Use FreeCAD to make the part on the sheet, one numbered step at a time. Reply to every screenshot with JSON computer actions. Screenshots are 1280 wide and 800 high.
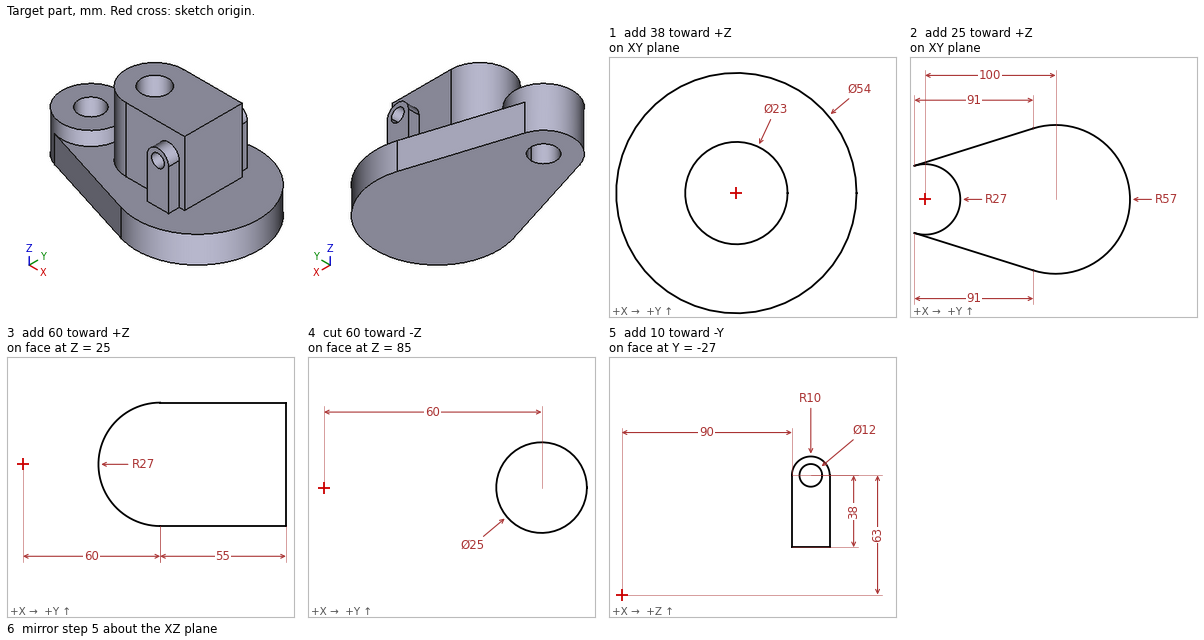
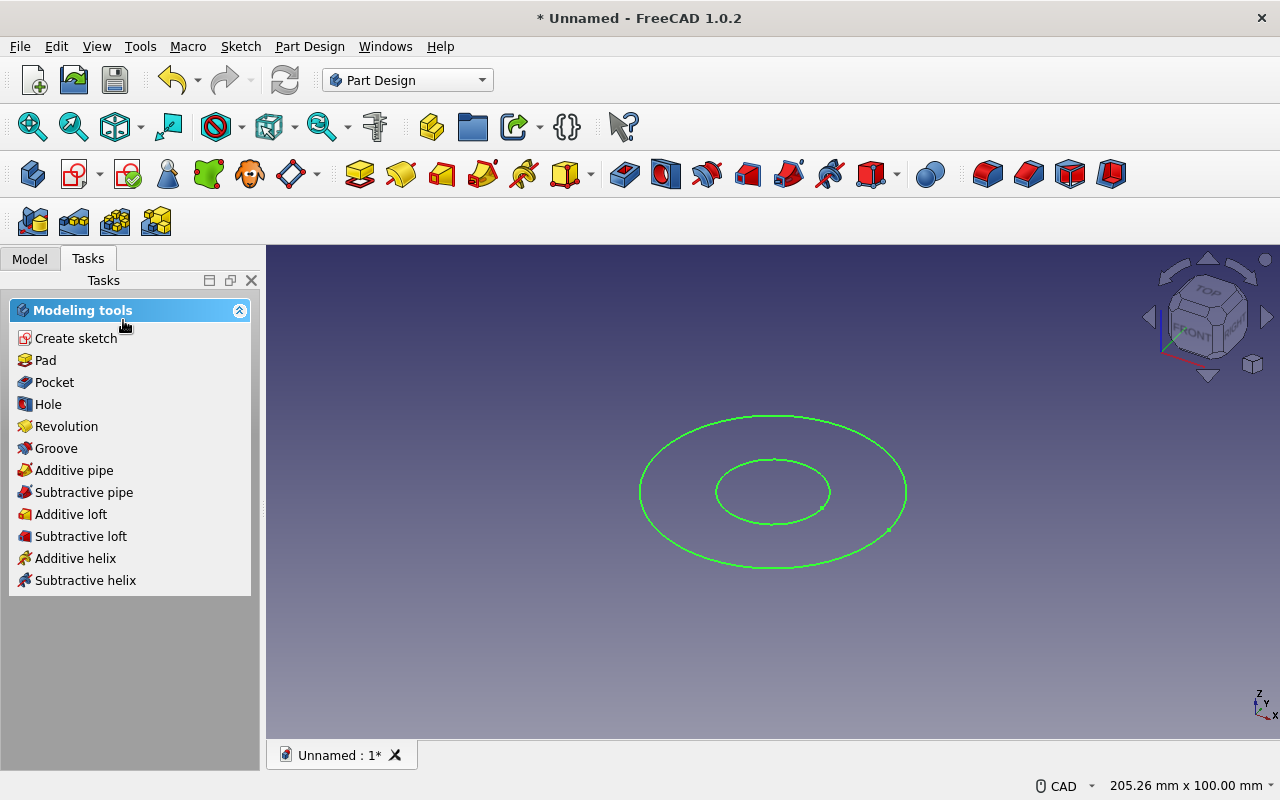
{"action": "left_click", "coordinate": [360, 174]}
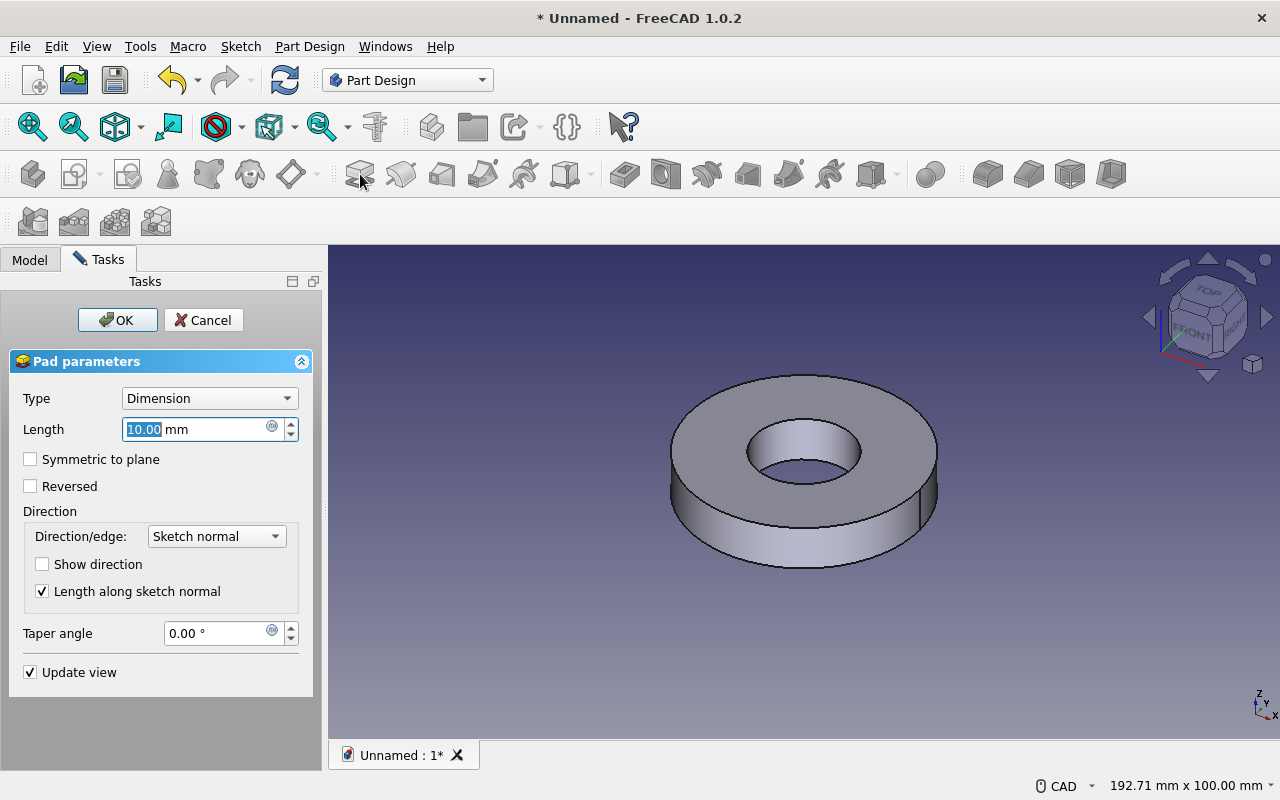
{"action": "type", "text": "38"}
{"action": "key", "text": "Tab"}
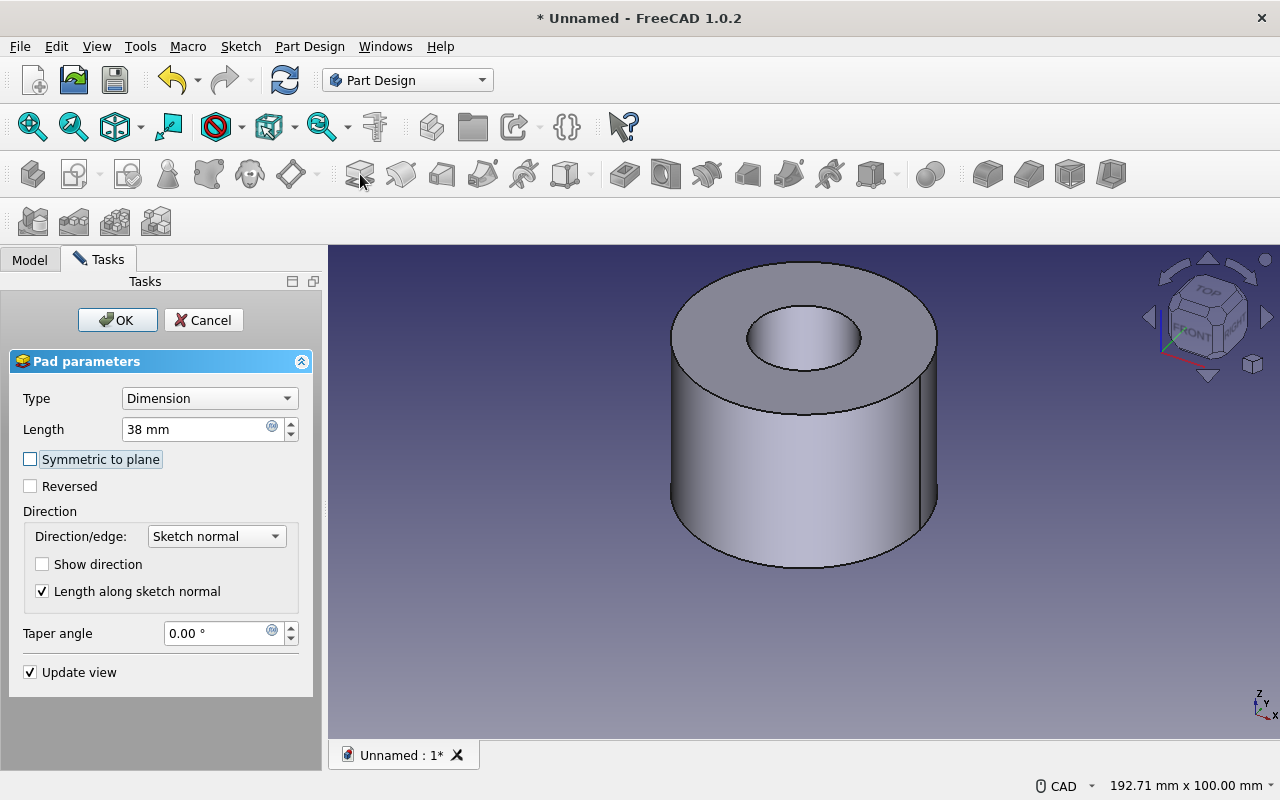
{"action": "left_click", "coordinate": [118, 320]}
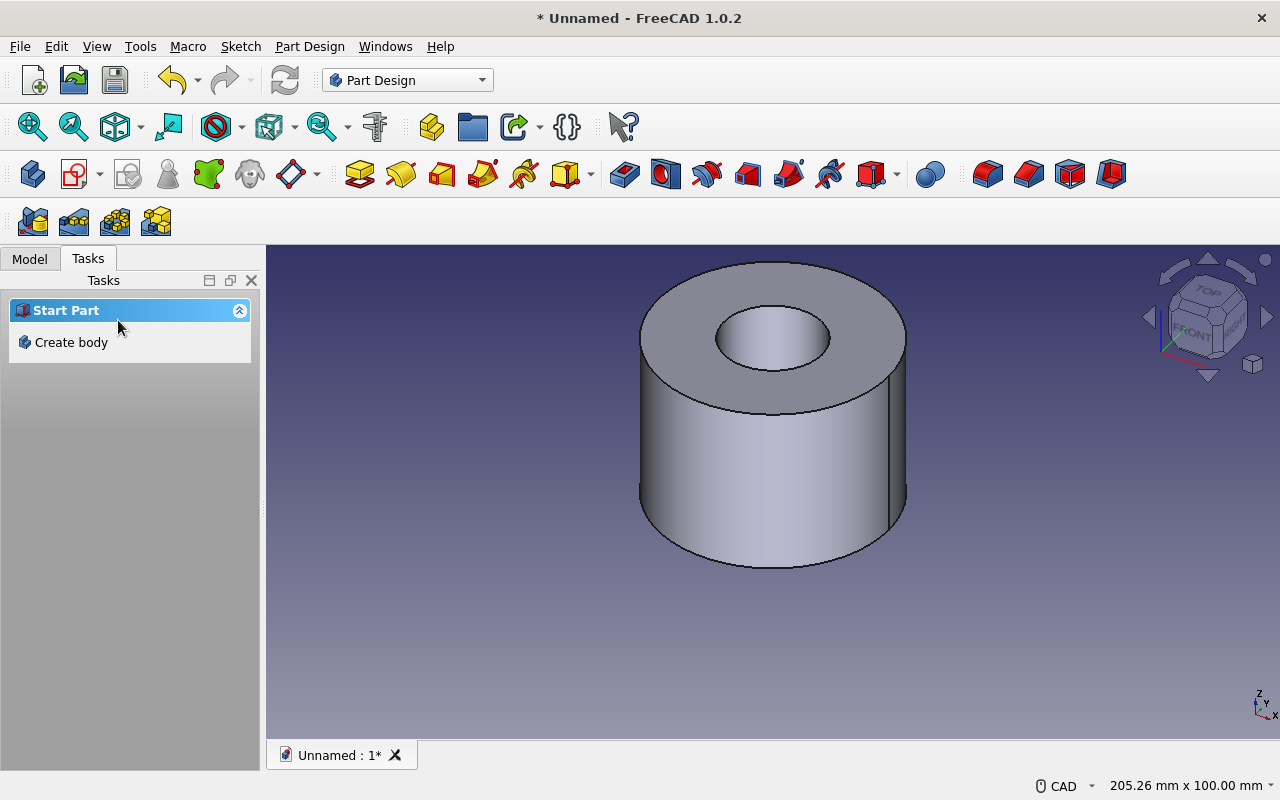
{"action": "left_click", "coordinate": [33, 128]}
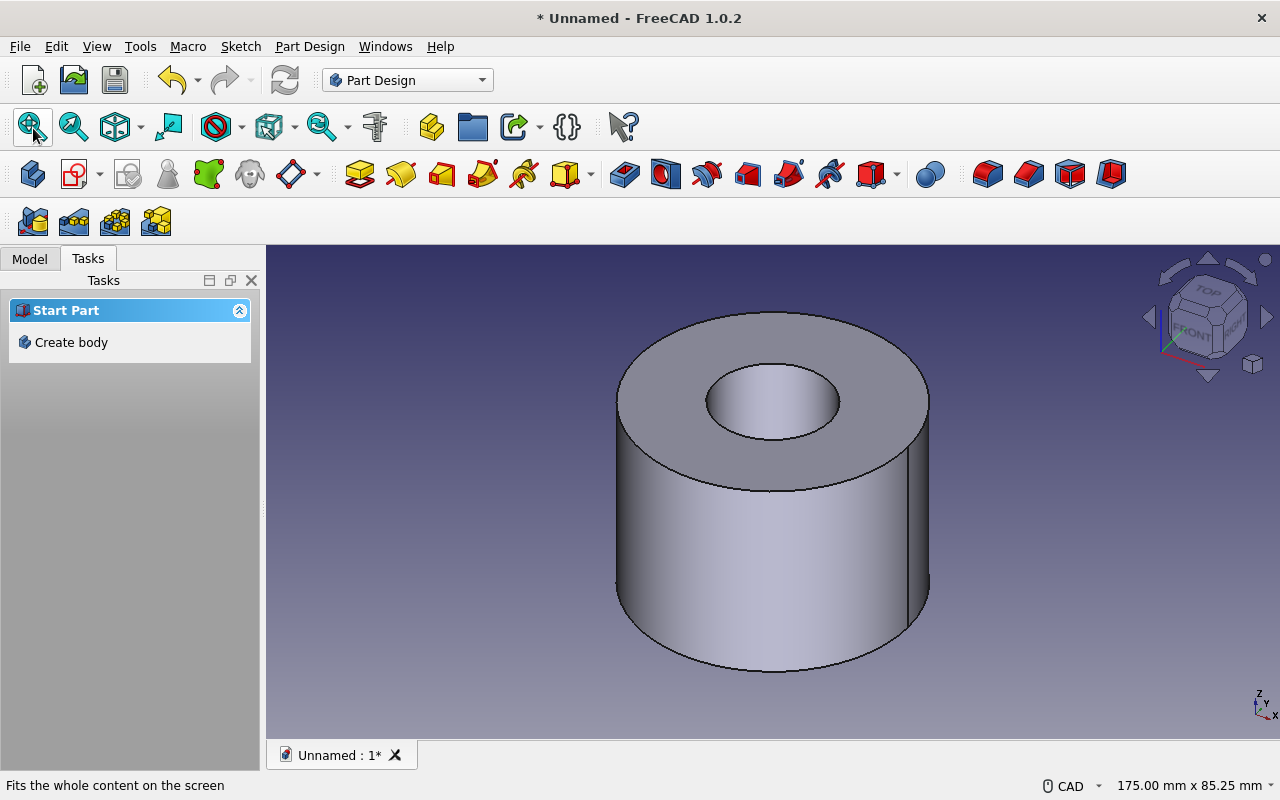
{"action": "left_click", "coordinate": [74, 174]}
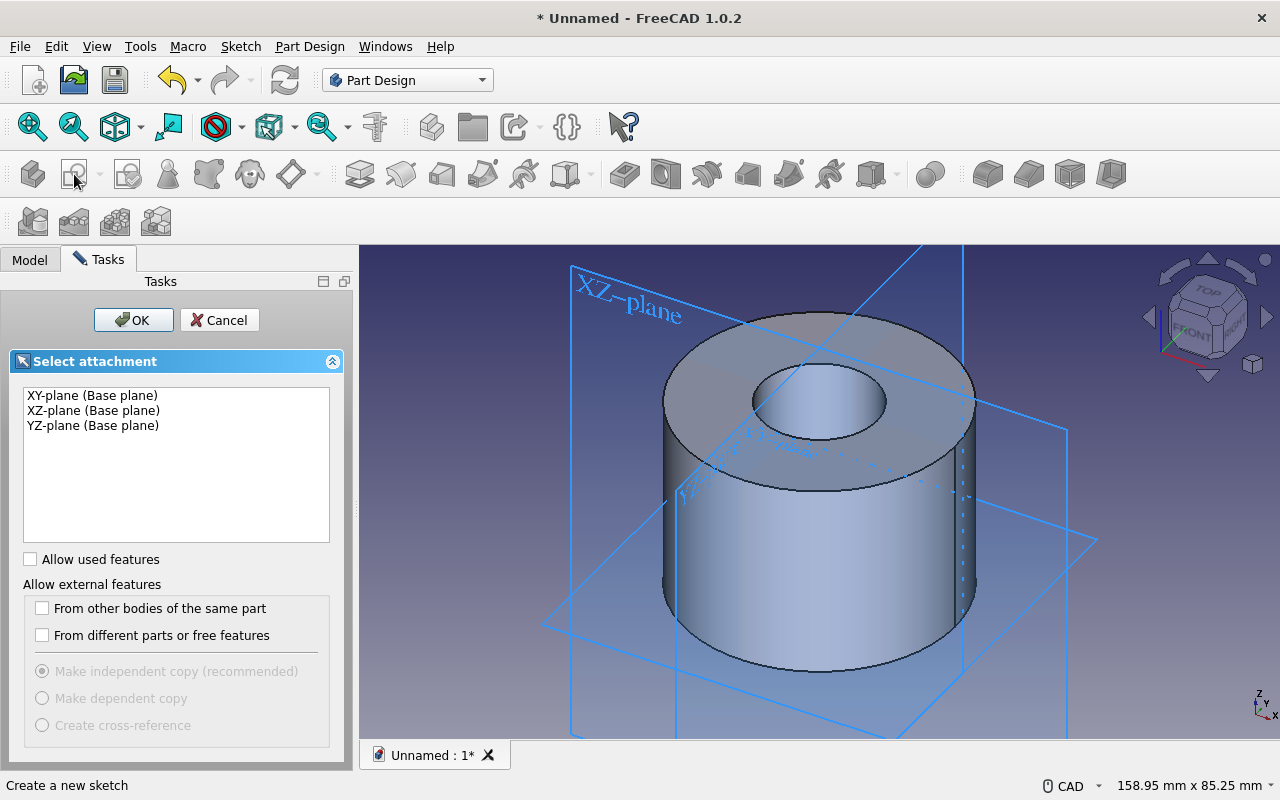
{"action": "left_click", "coordinate": [84, 396]}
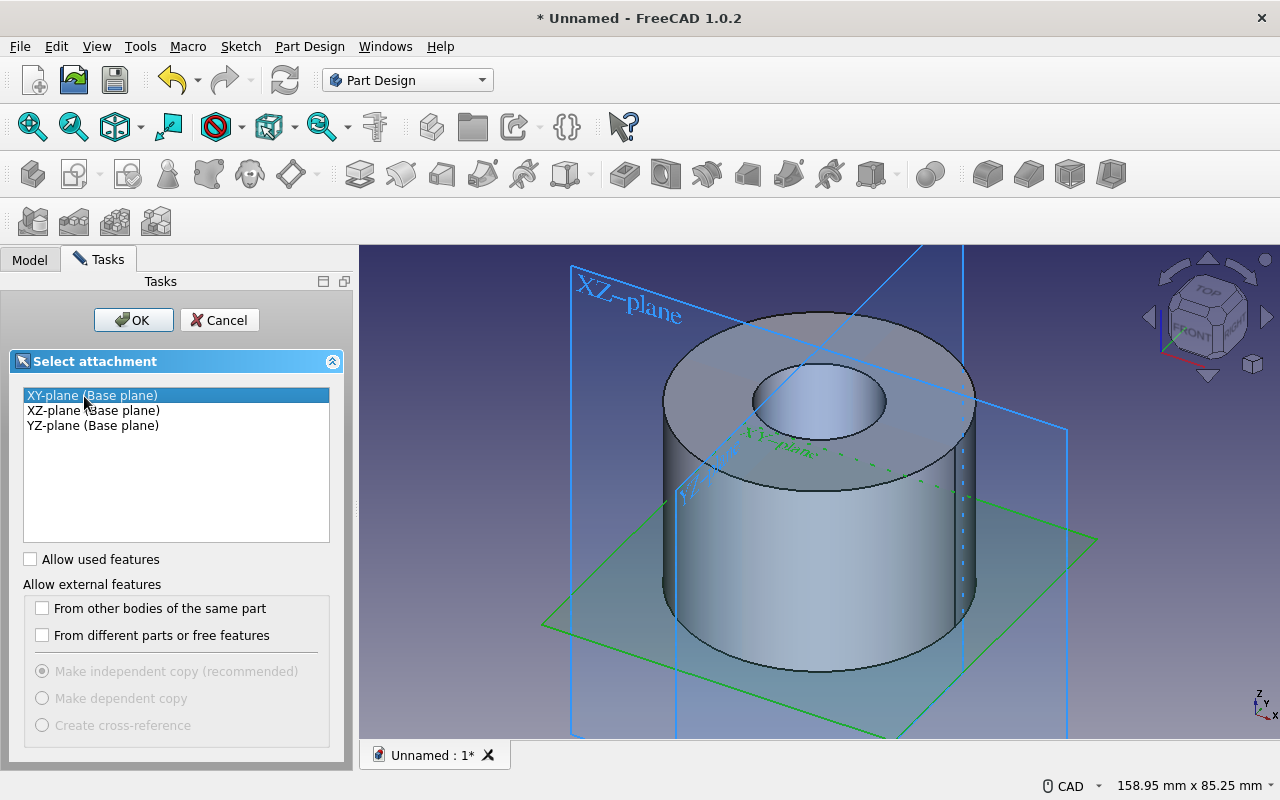
{"action": "left_click", "coordinate": [134, 320]}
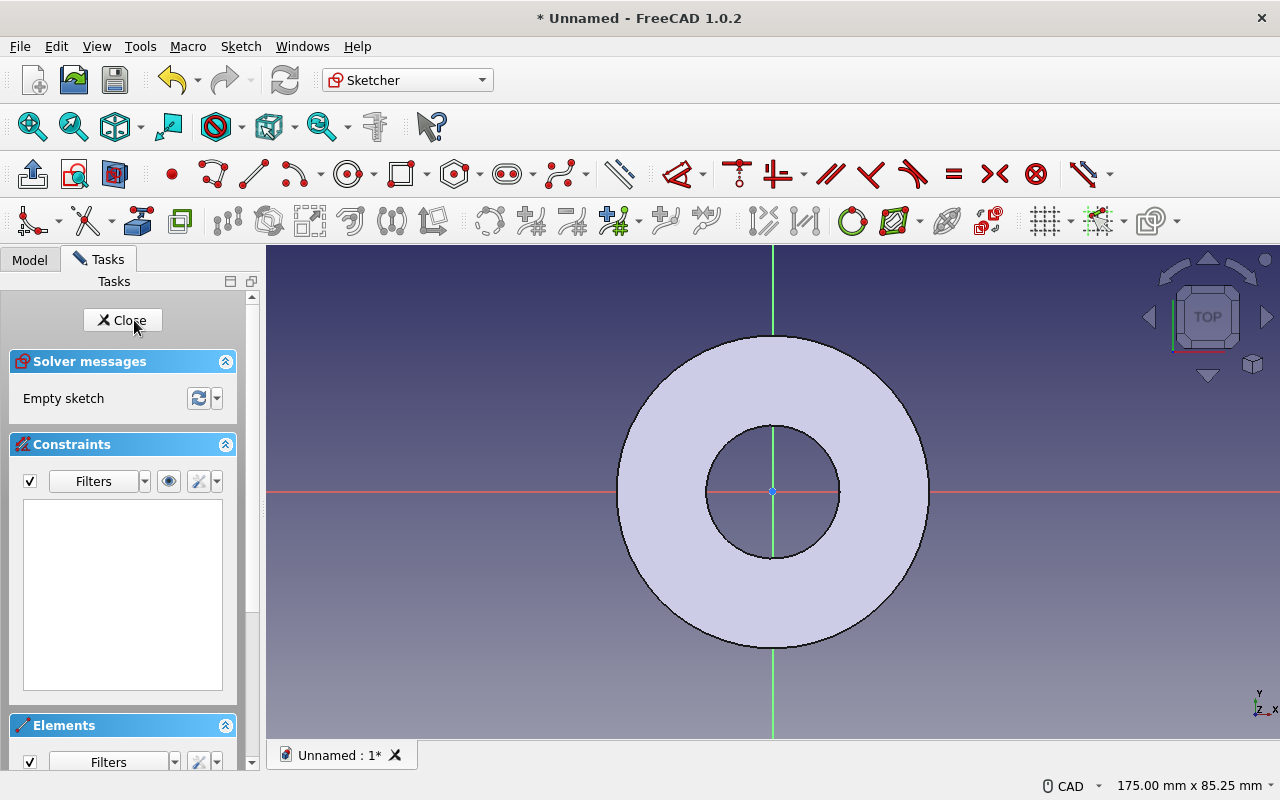
{"action": "key", "text": "q s"}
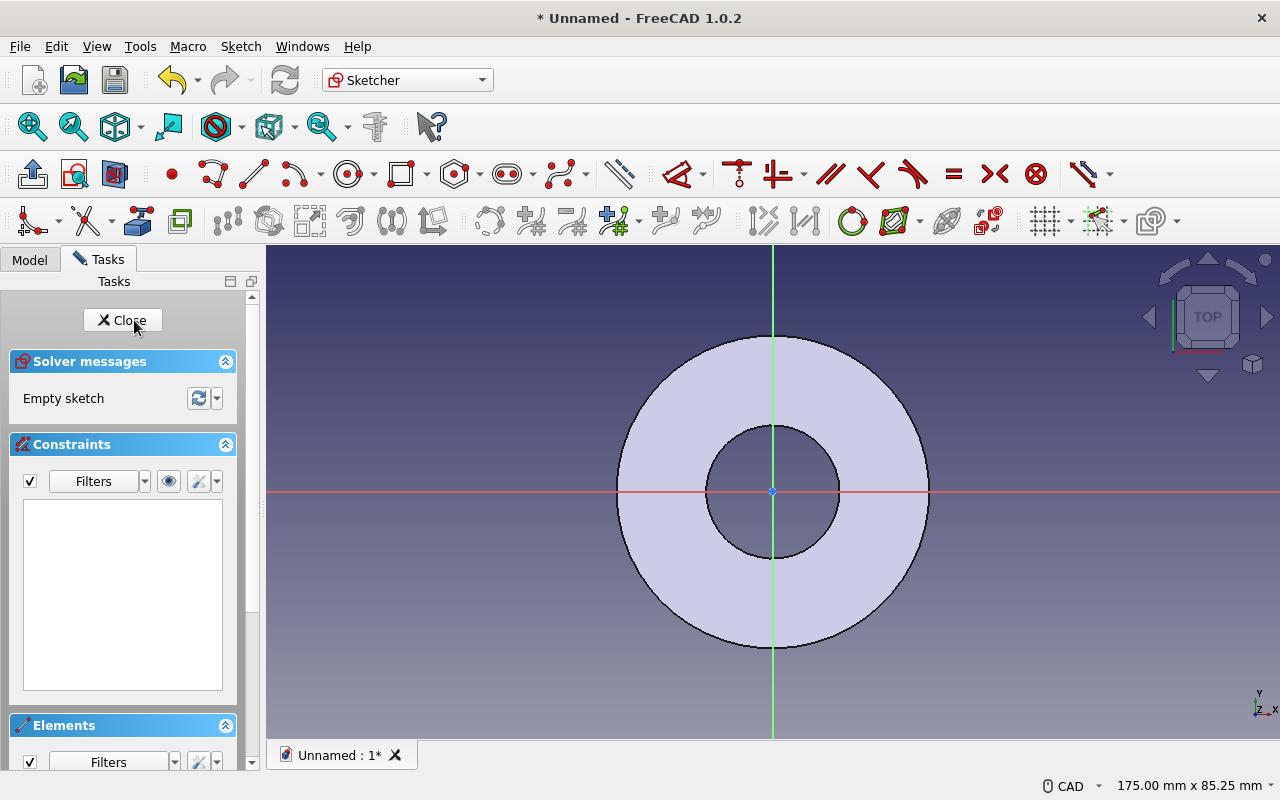
{"action": "scroll", "coordinate": [297, 492], "scroll_direction": "down", "scroll_amount": 4}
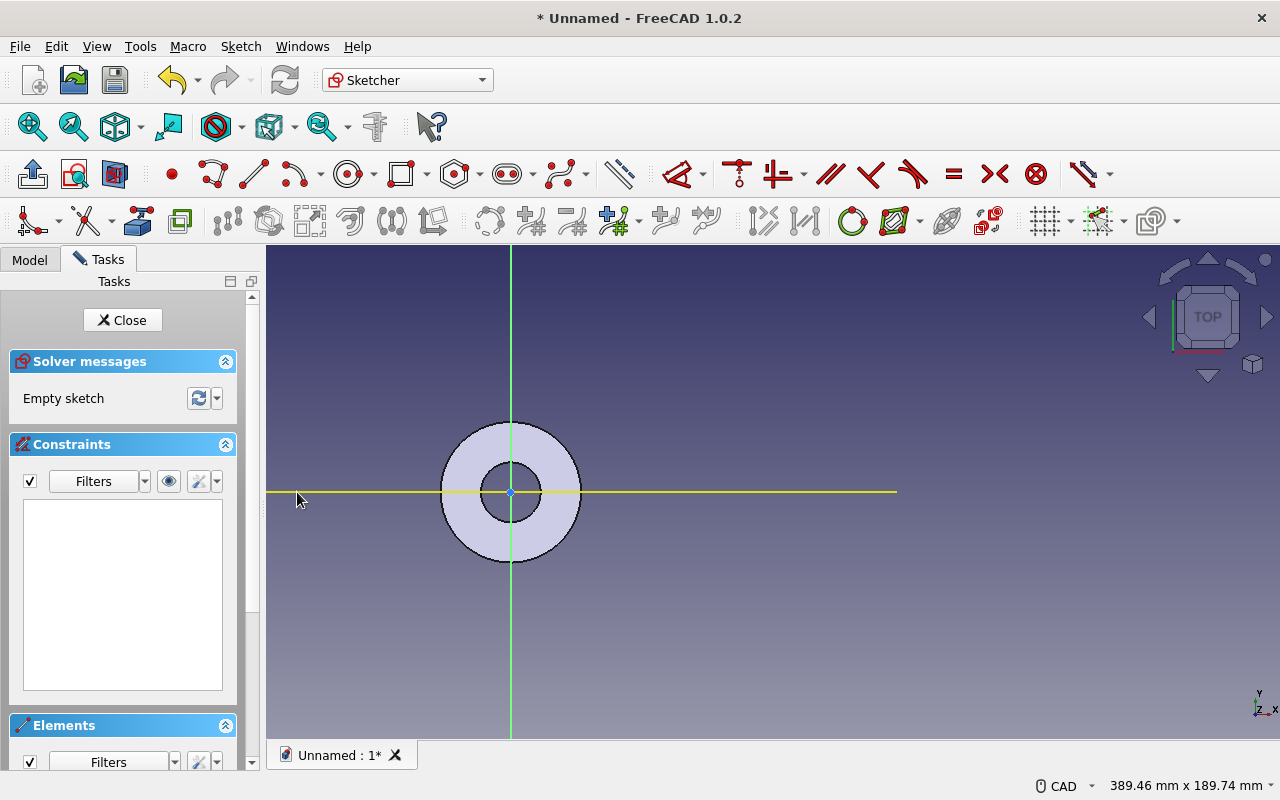
{"action": "left_click", "coordinate": [254, 174]}